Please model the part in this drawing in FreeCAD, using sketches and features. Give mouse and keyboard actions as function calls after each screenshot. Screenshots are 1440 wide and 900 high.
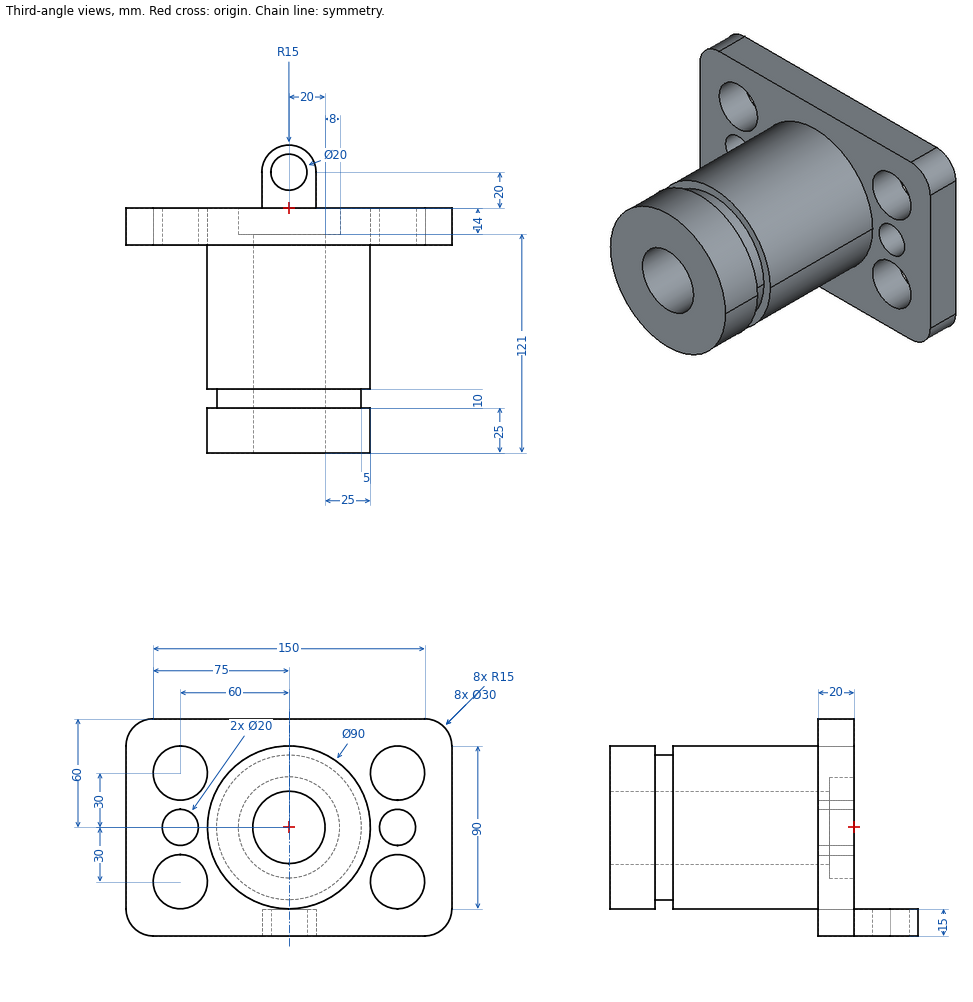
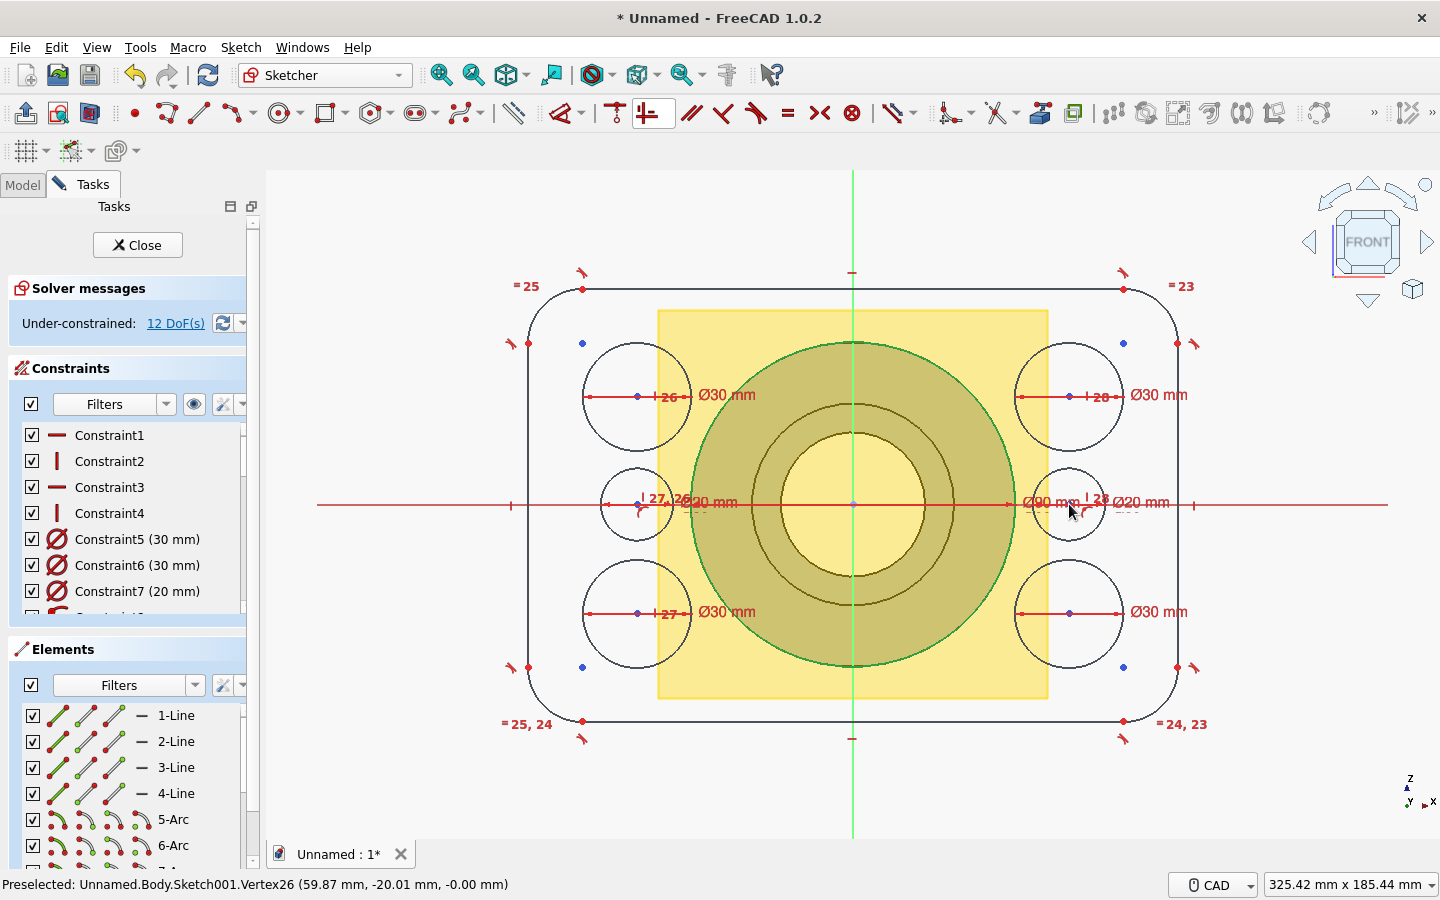
click(1069, 504)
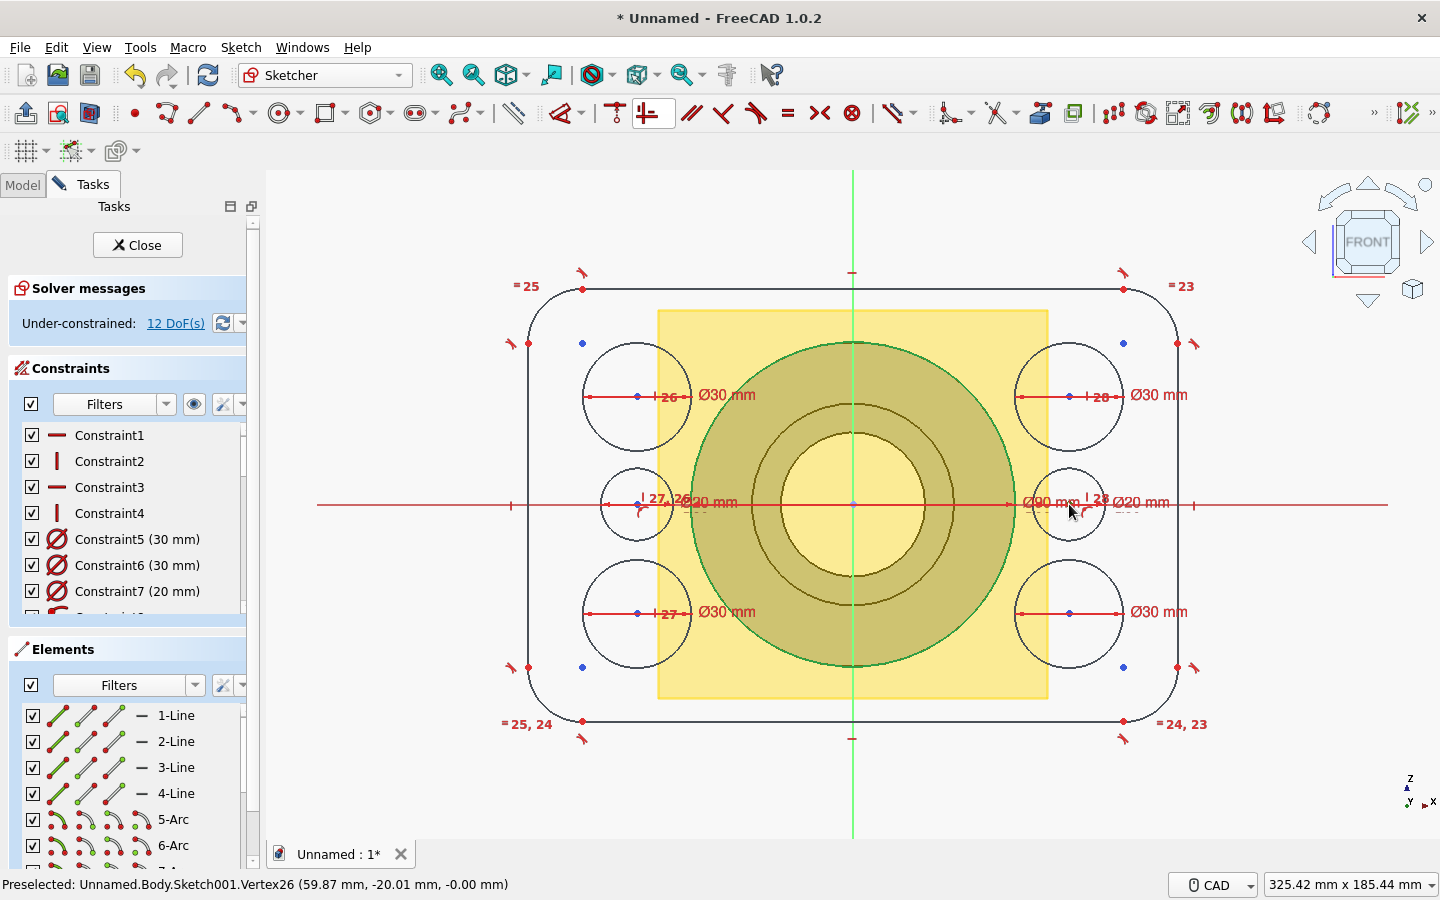
click(1069, 614)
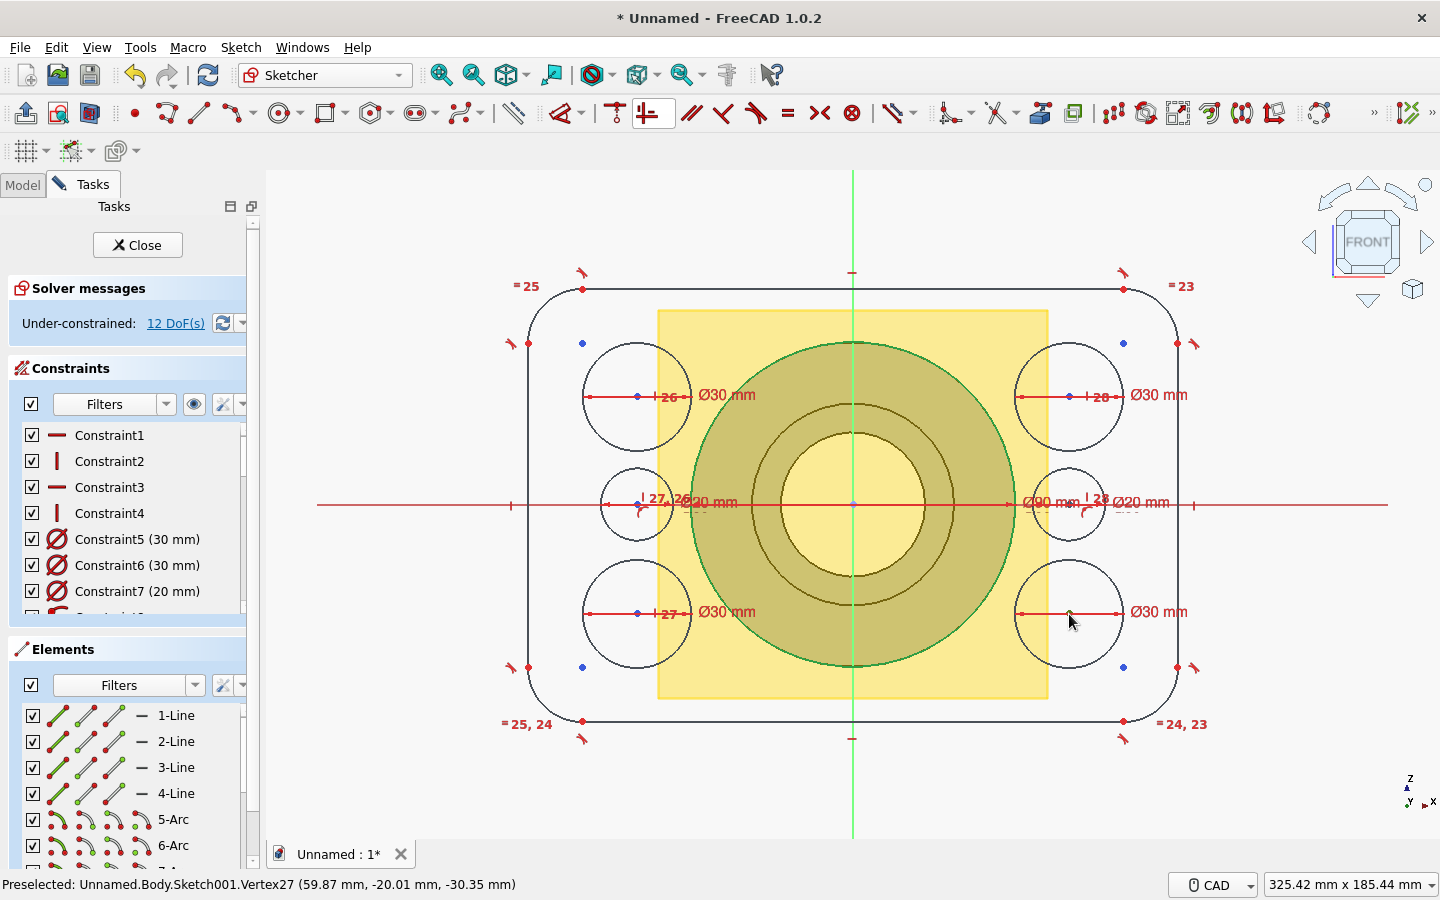
key(v)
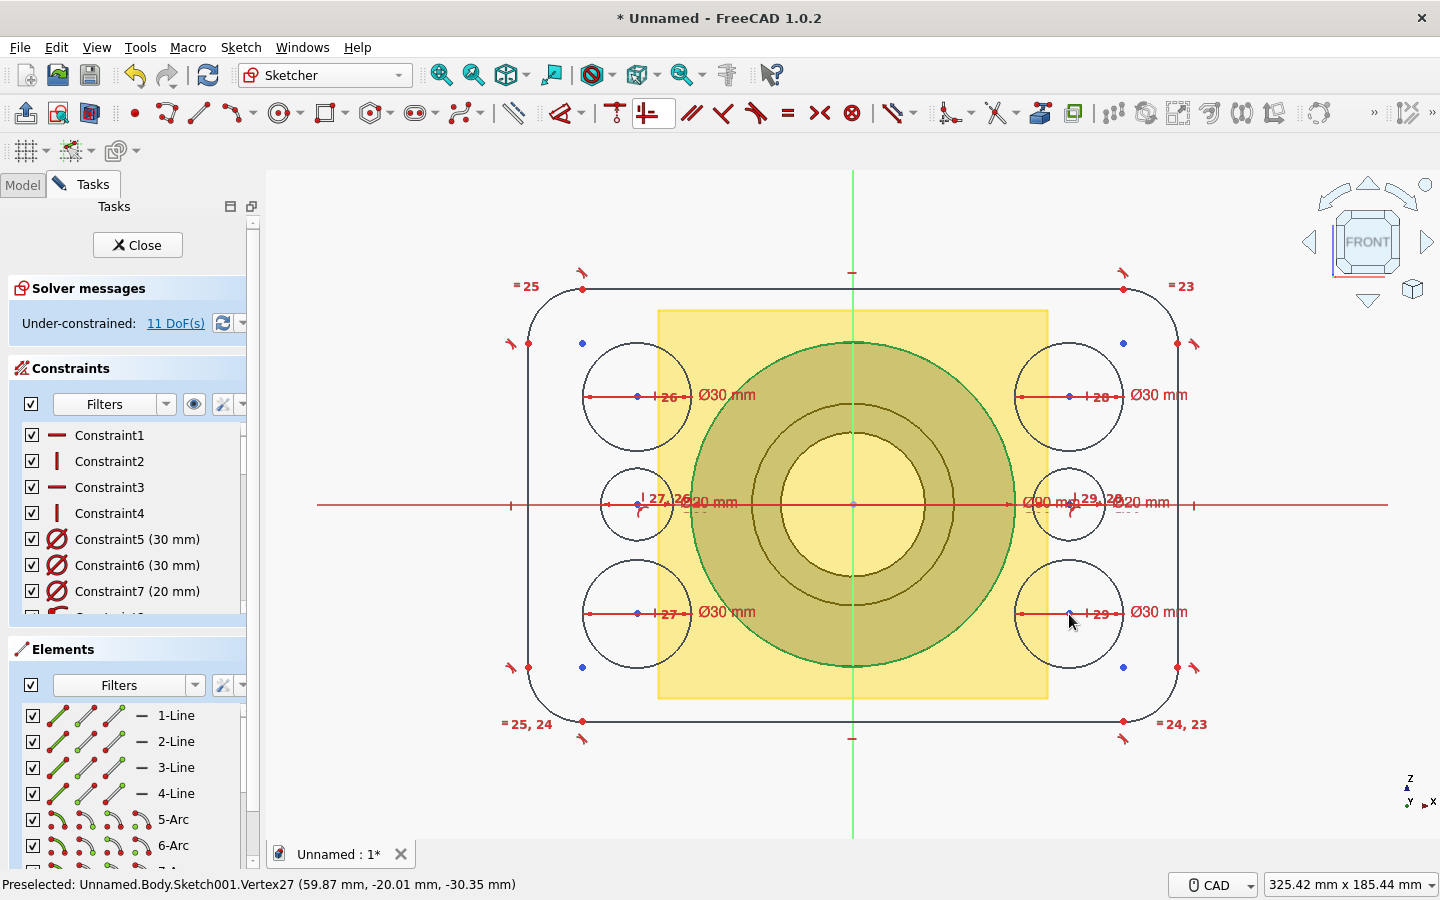
click(637, 397)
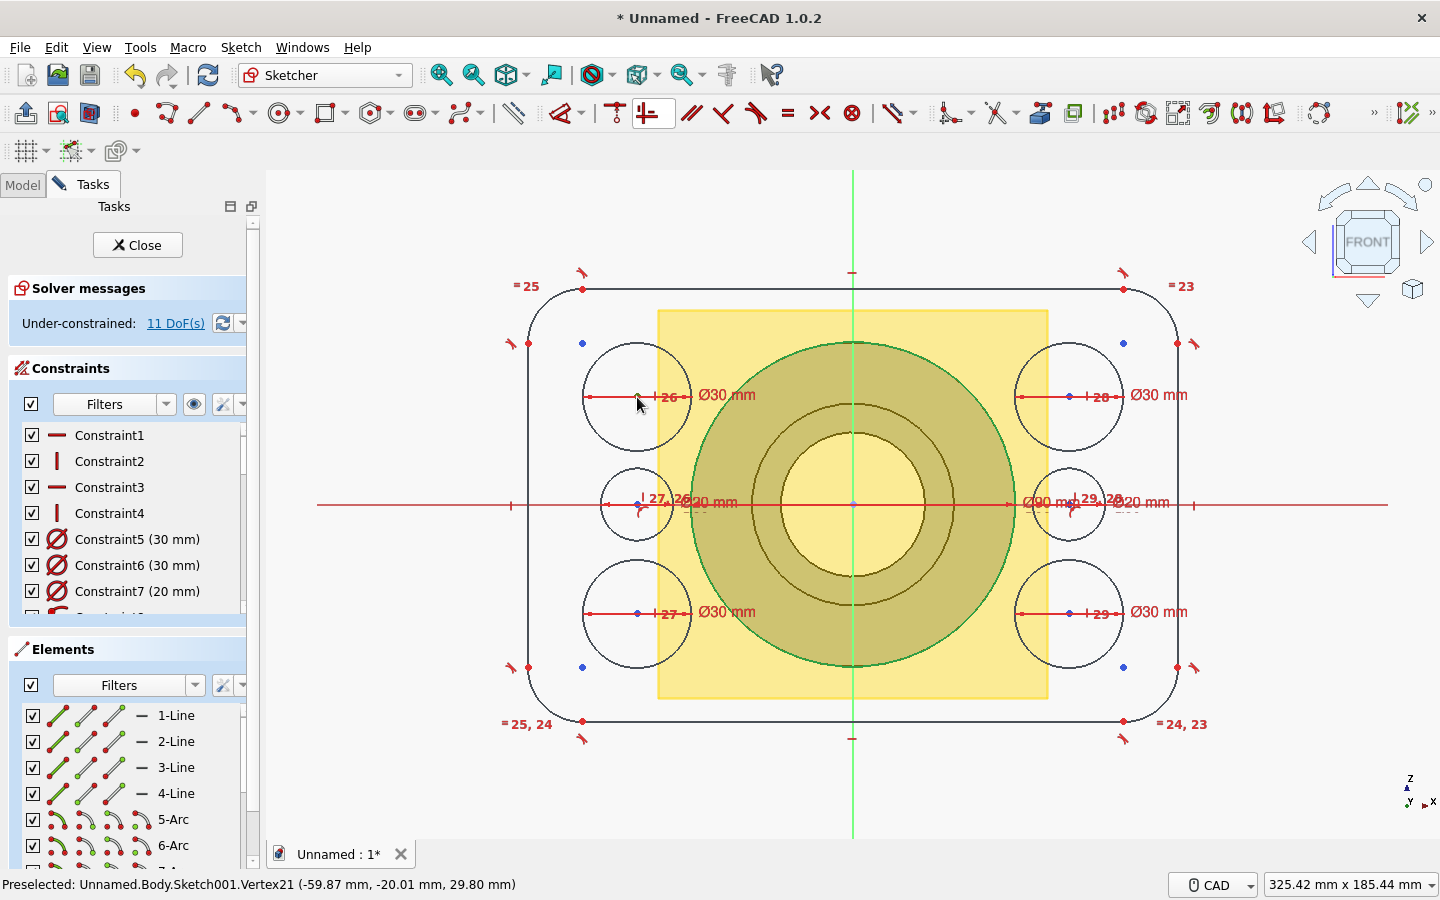
click(1069, 397)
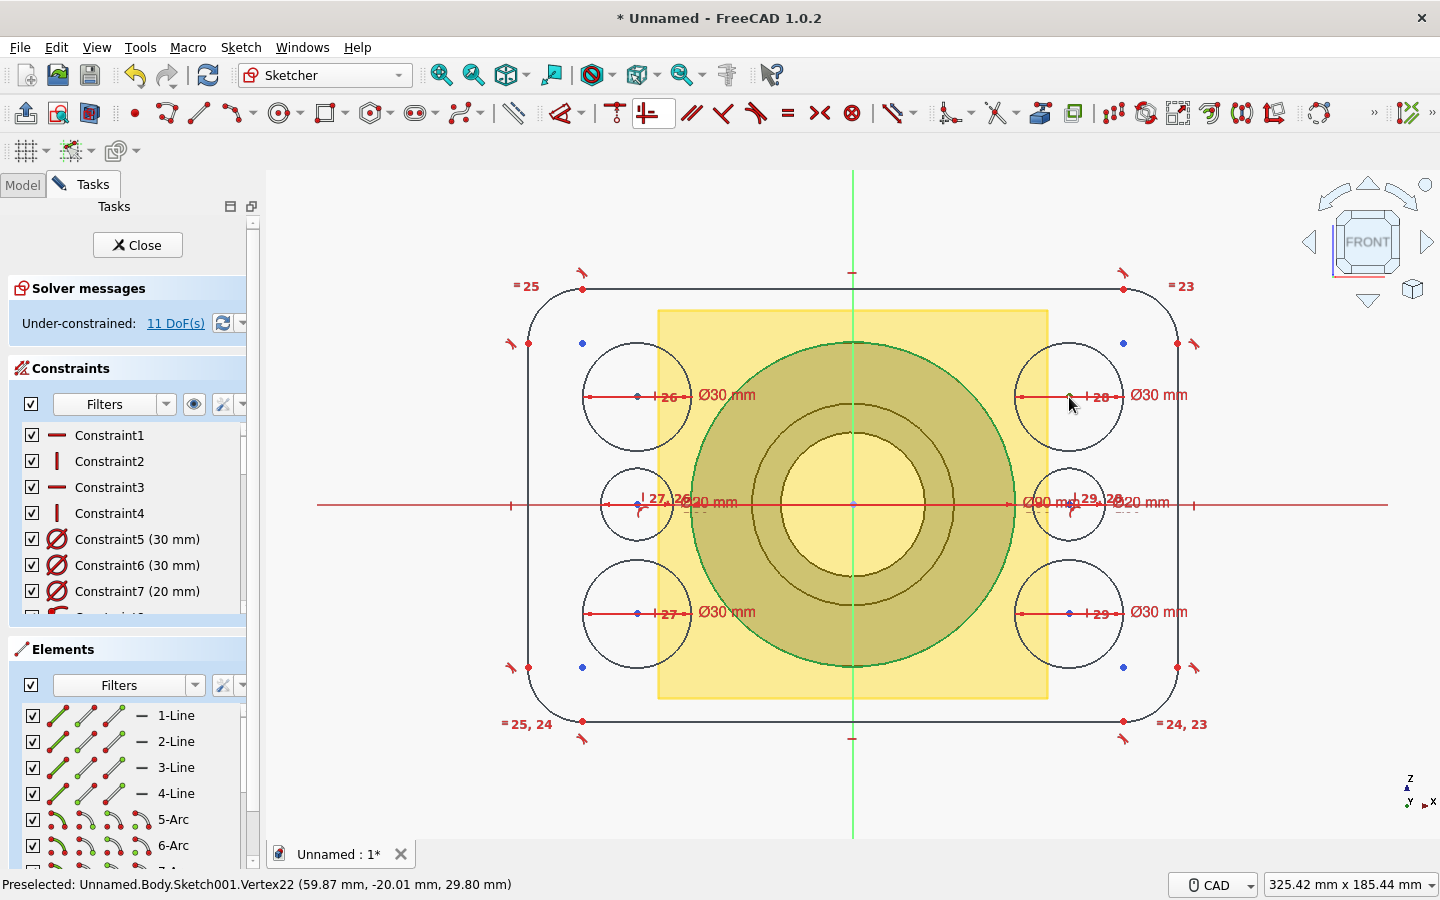
click(853, 767)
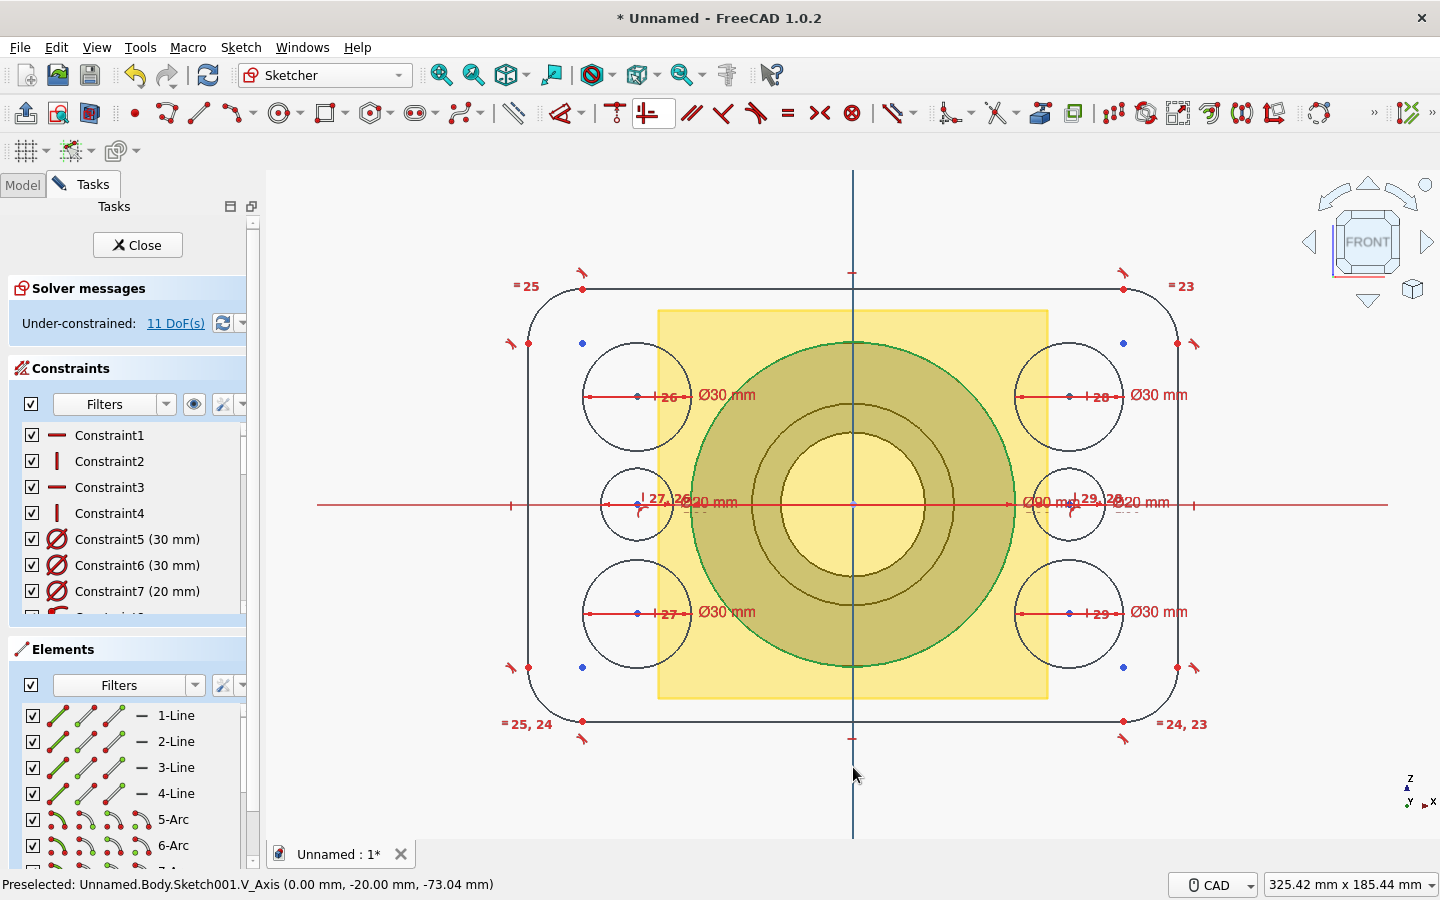
key(s)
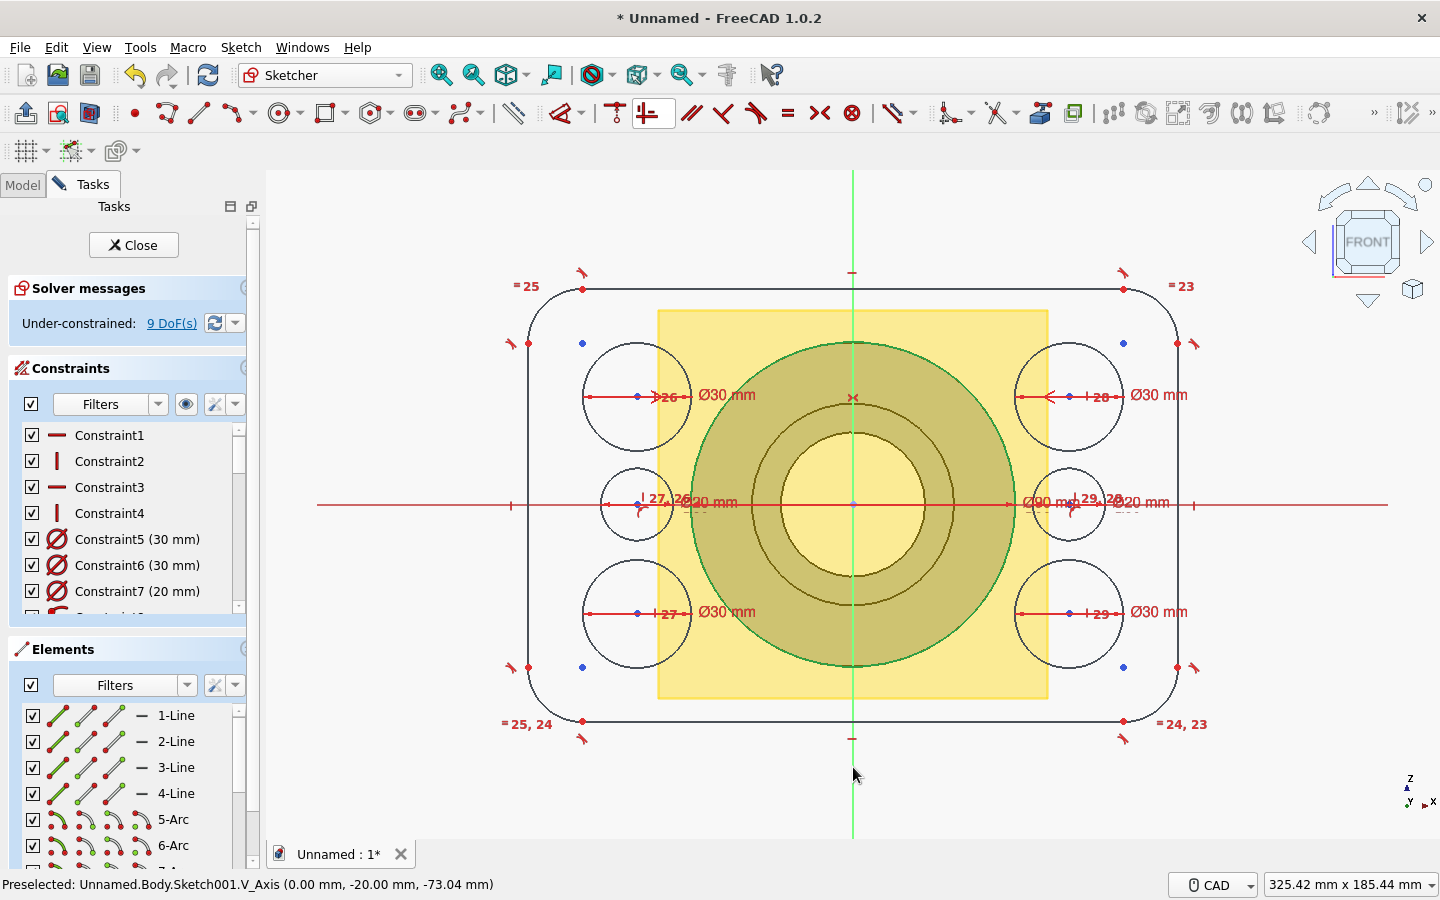
click(560, 114)